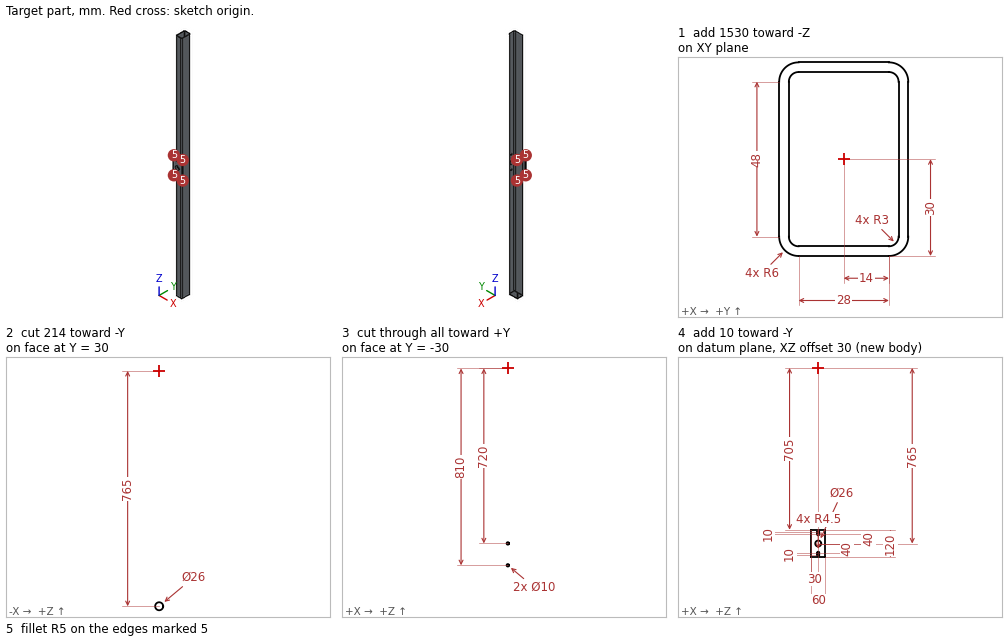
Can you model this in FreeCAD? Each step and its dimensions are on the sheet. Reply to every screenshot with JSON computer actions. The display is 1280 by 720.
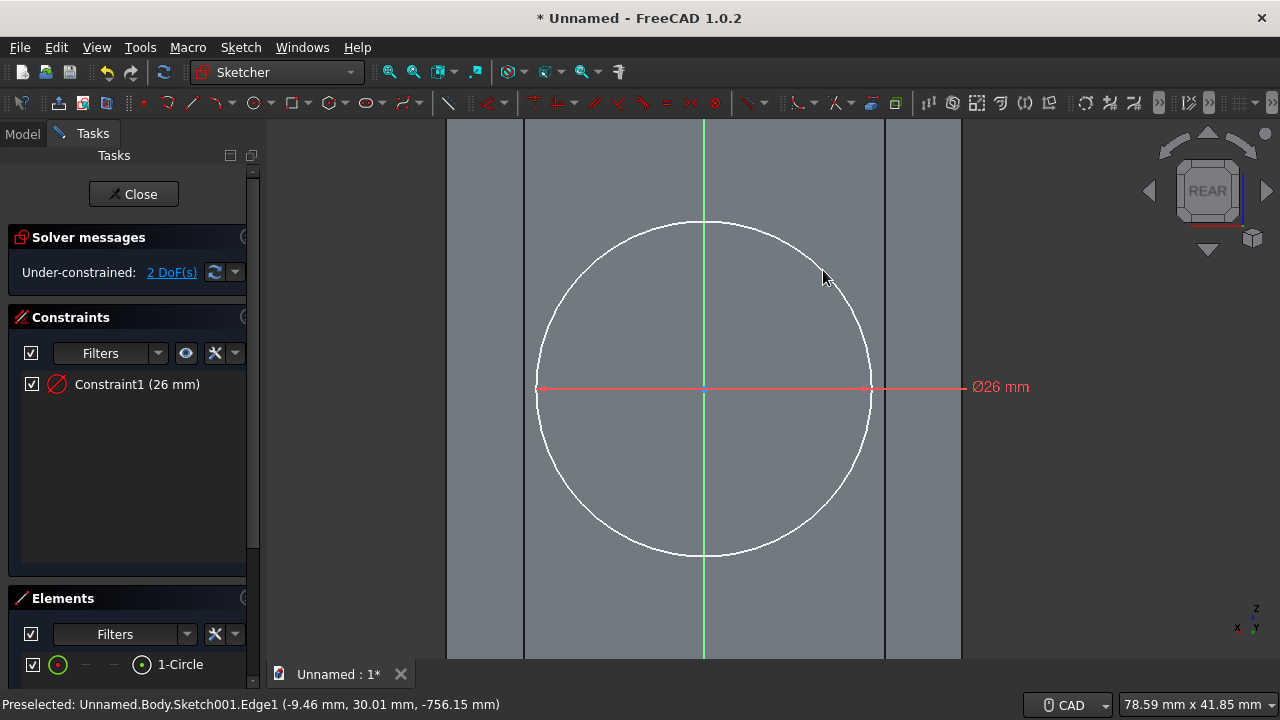
{"action": "left_click", "coordinate": [704, 389]}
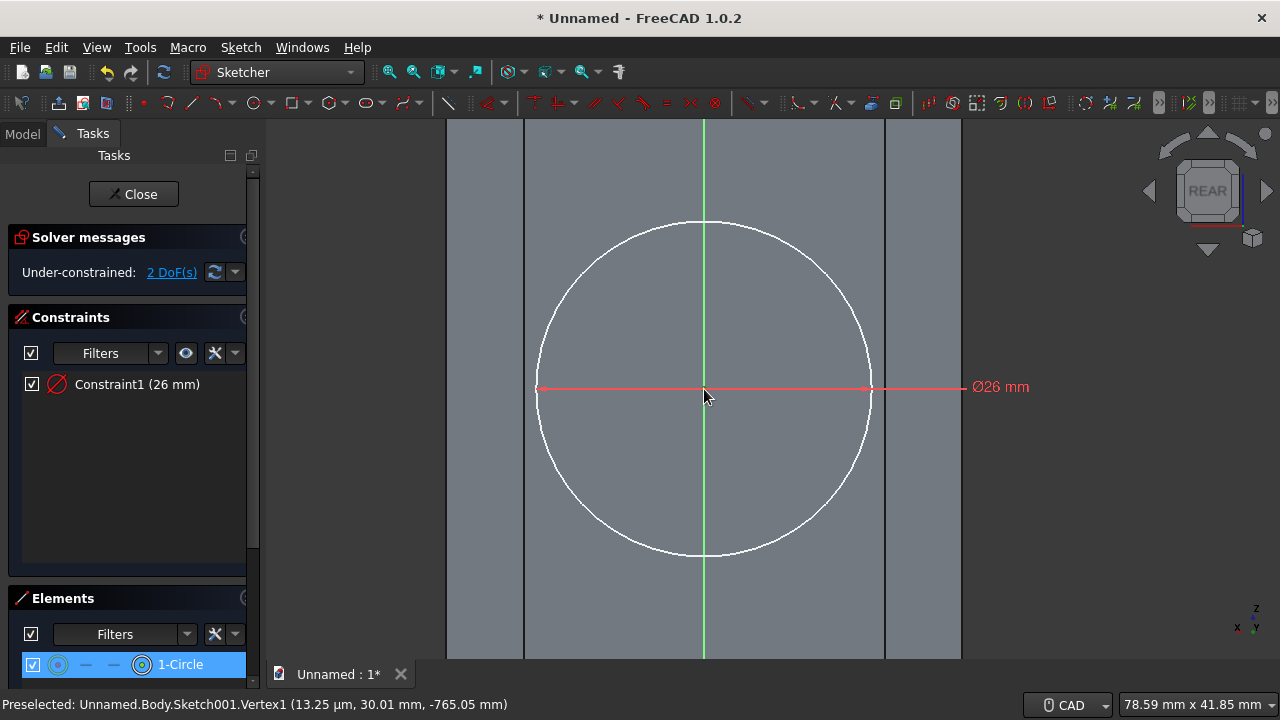
{"action": "left_click", "coordinate": [704, 596]}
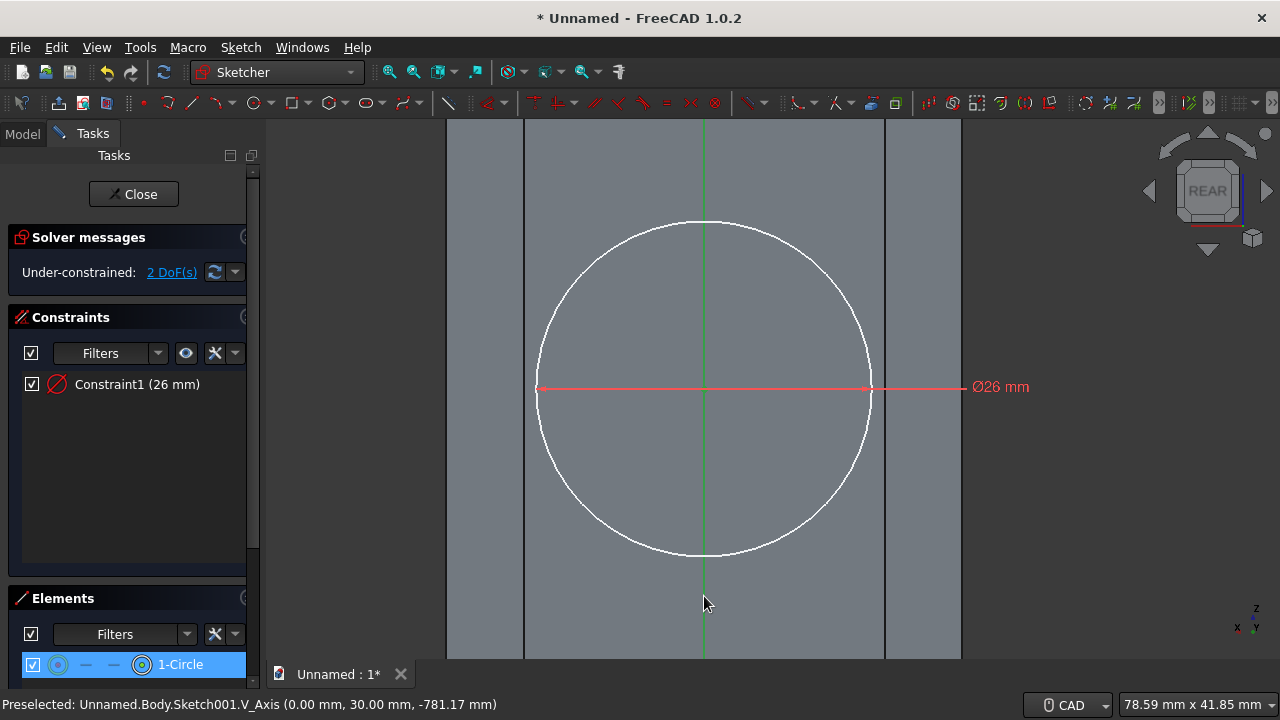
{"action": "left_click", "coordinate": [534, 104]}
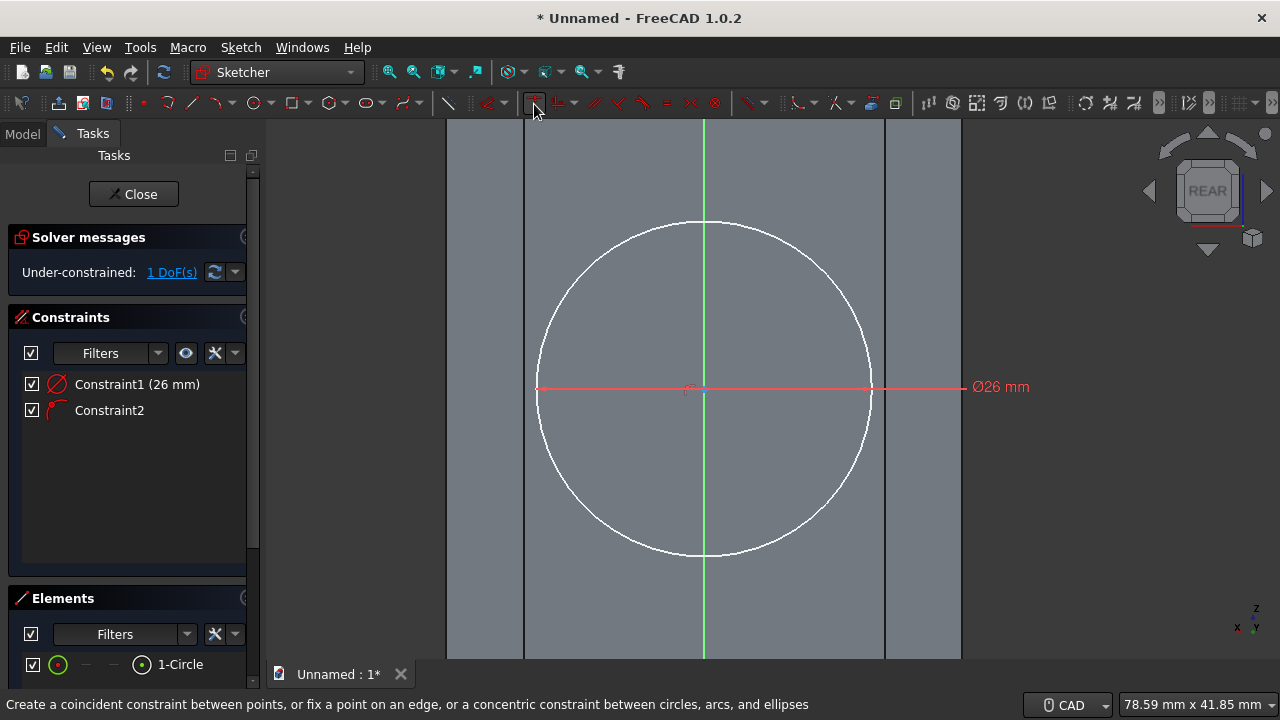
{"action": "left_click", "coordinate": [488, 104]}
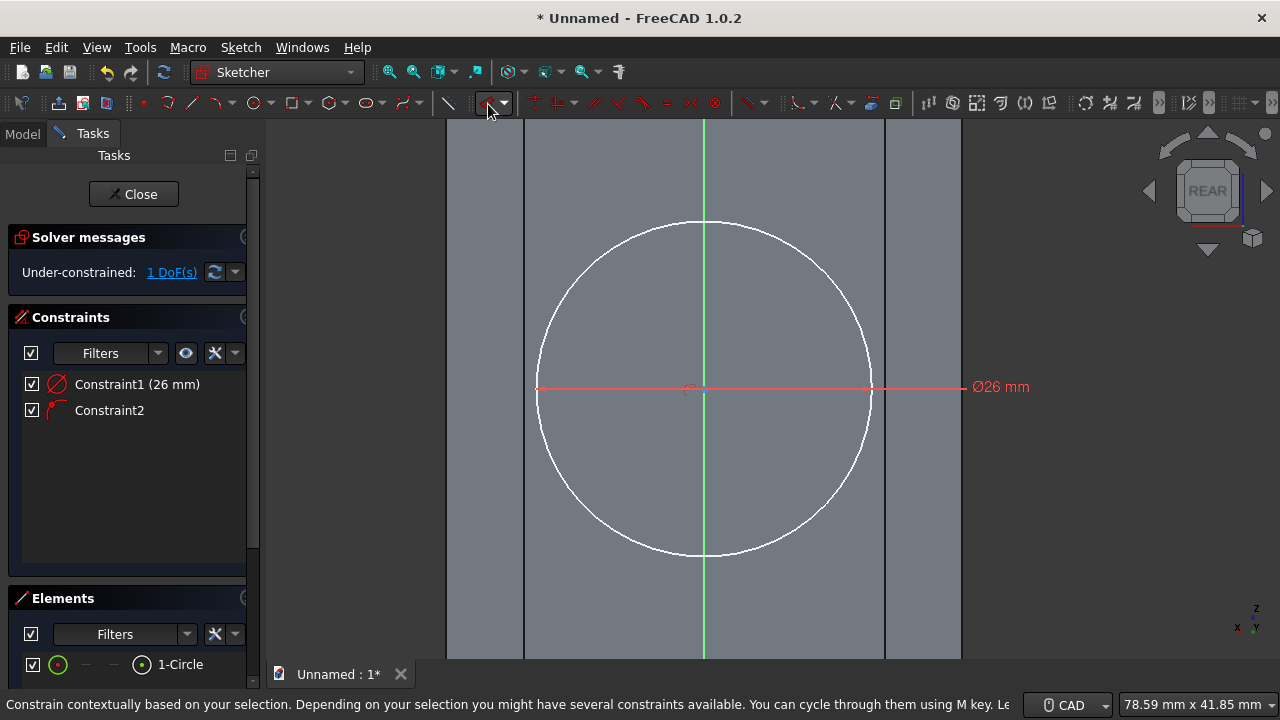
{"action": "left_click", "coordinate": [704, 389]}
{"action": "left_click", "coordinate": [738, 268]}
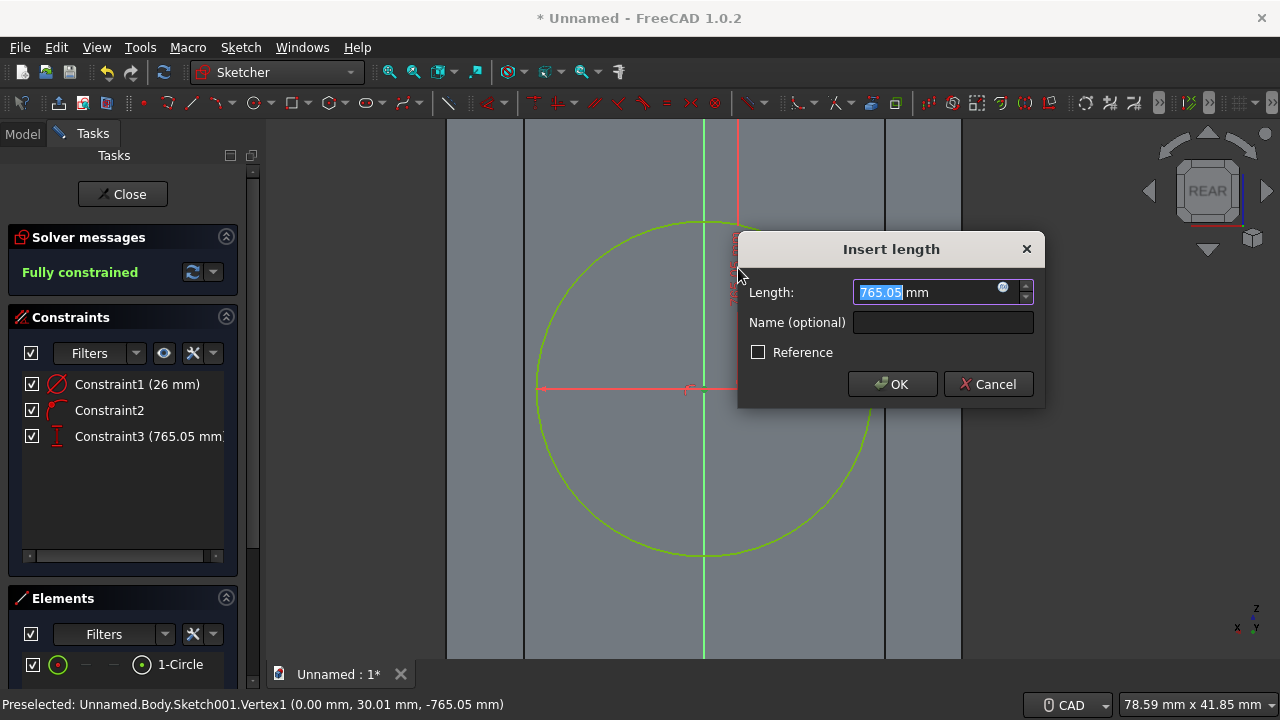
{"action": "type", "text": "765"}
{"action": "key", "text": "Return"}
{"action": "key", "text": "Escape"}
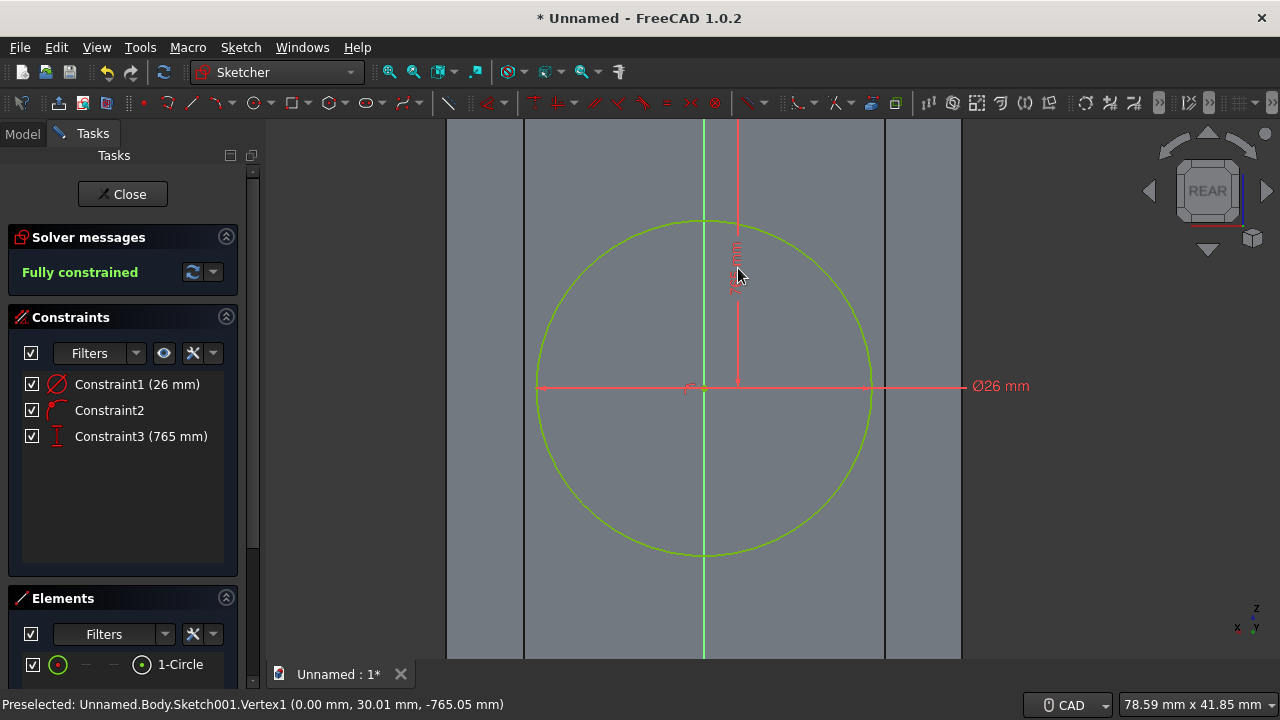
{"action": "left_click", "coordinate": [123, 194]}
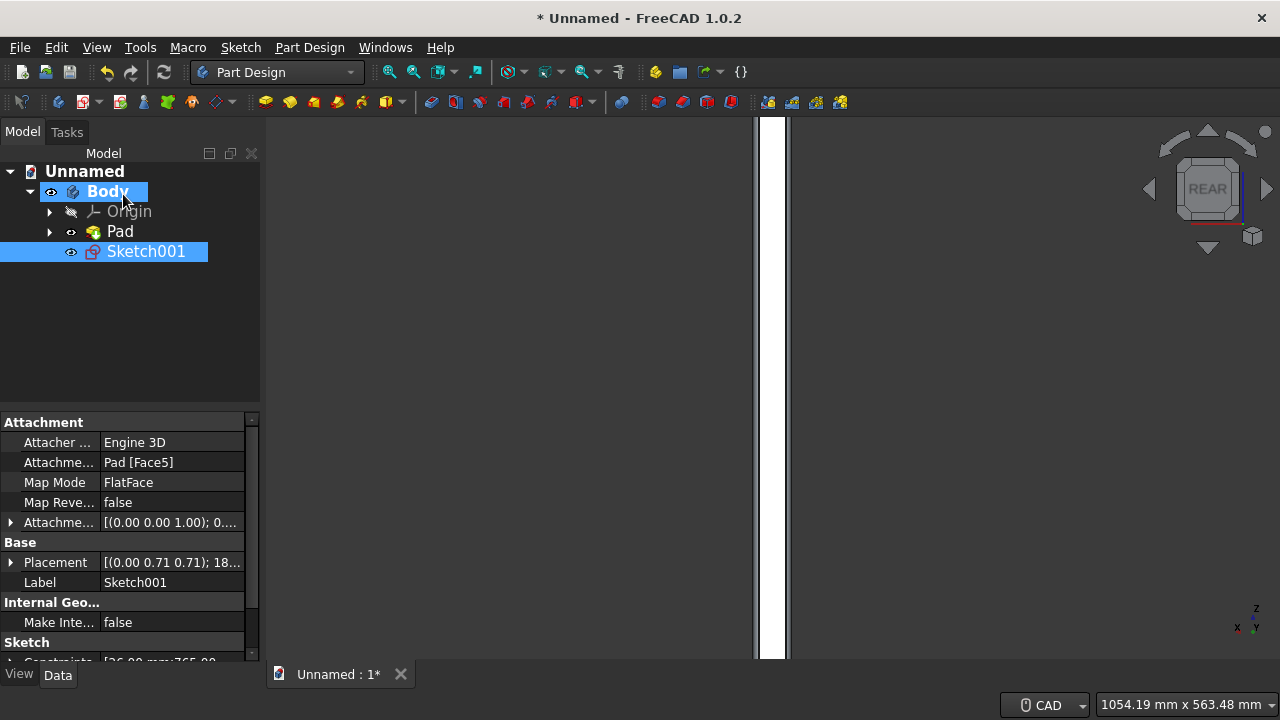
{"action": "left_click", "coordinate": [432, 102]}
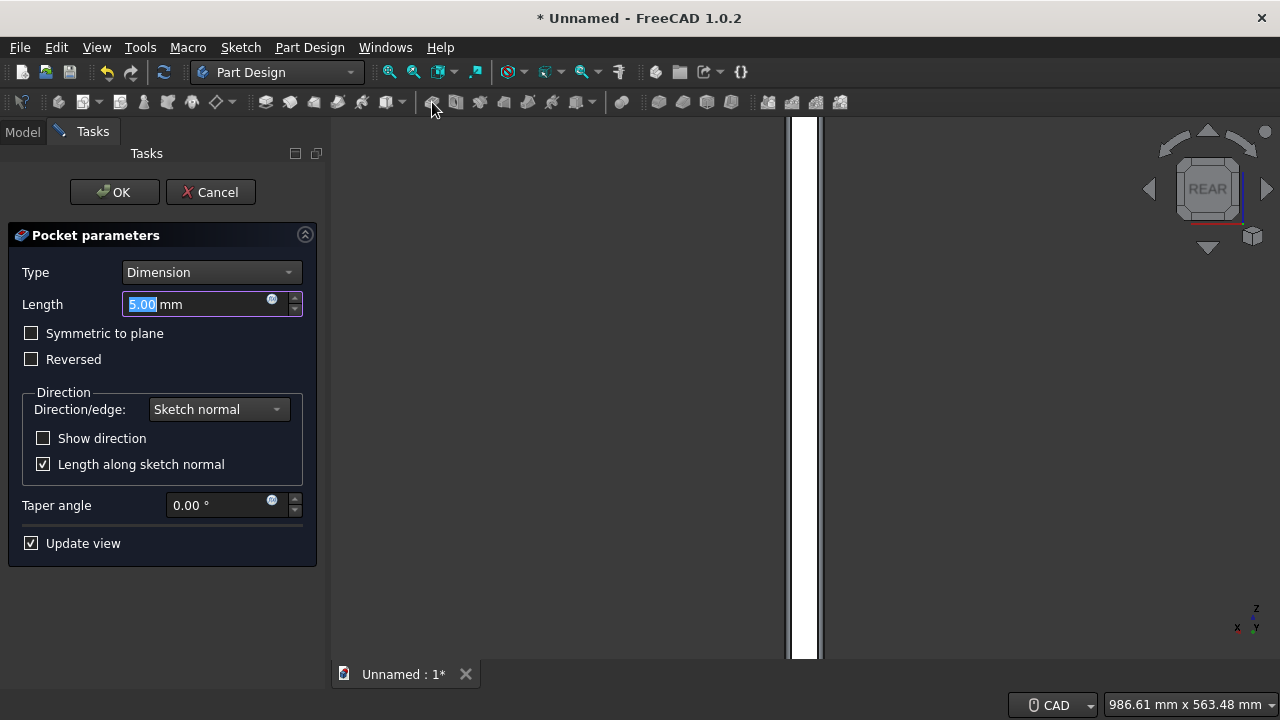
{"action": "type", "text": "214"}
{"action": "key", "text": "Tab"}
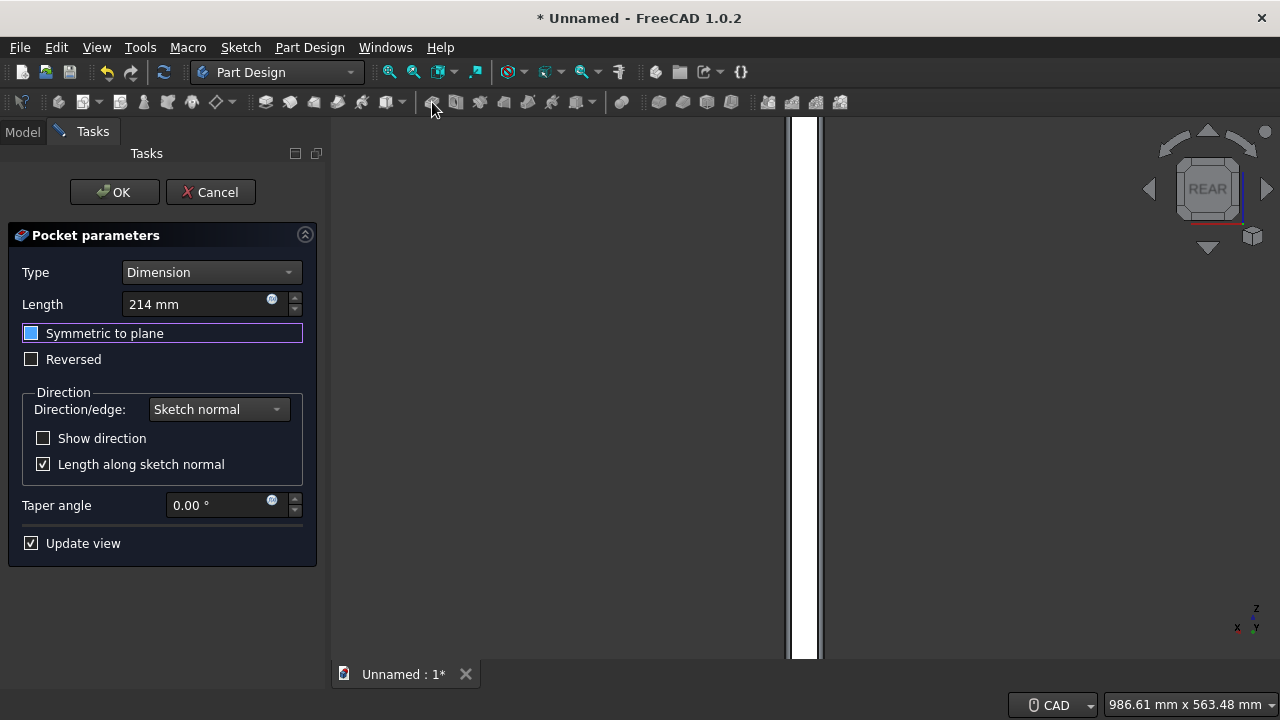
{"action": "left_click", "coordinate": [115, 192]}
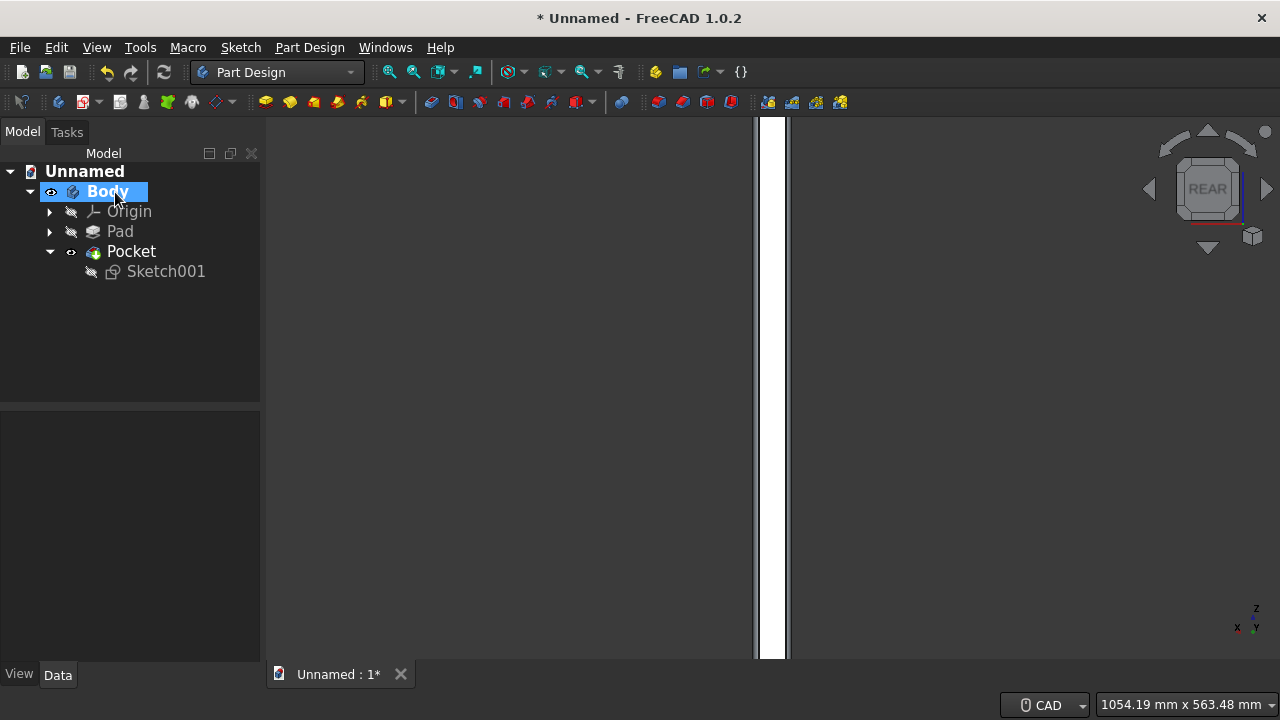
{"action": "left_click", "coordinate": [390, 72]}